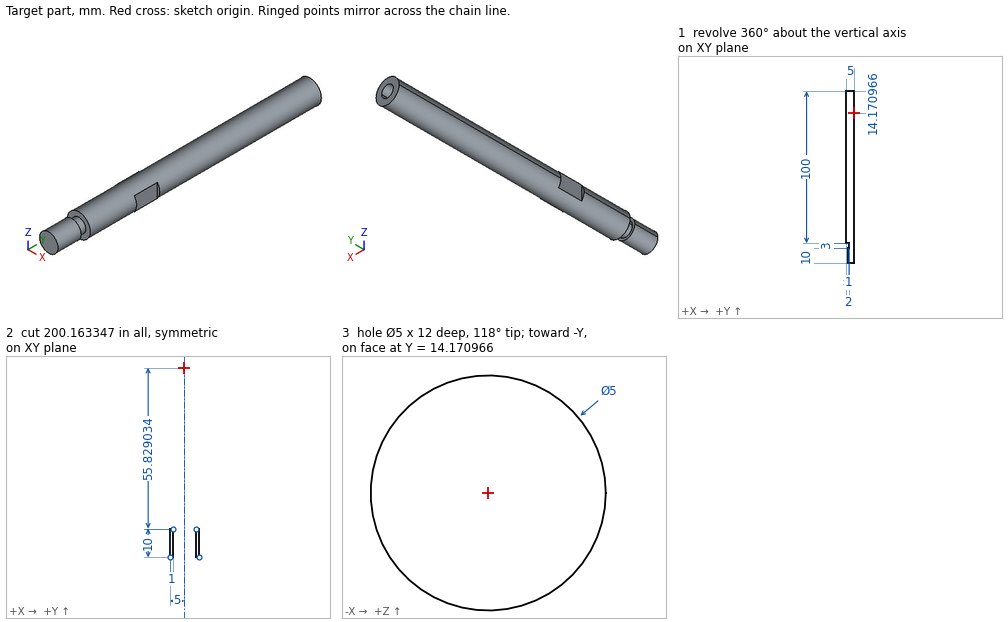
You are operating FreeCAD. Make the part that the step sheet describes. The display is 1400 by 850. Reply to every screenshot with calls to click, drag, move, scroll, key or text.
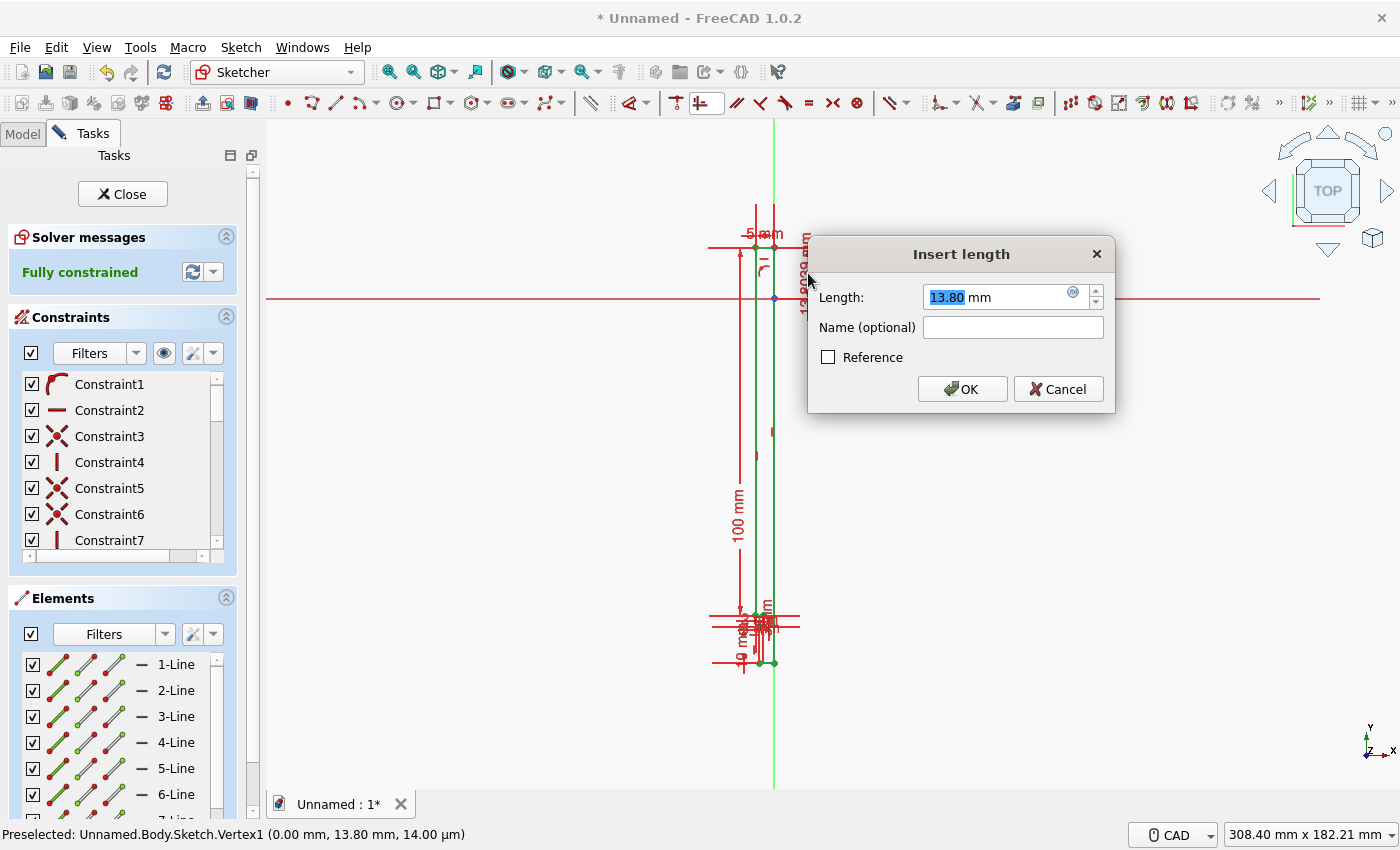
text(14.170966)
key(Return)
key(Escape)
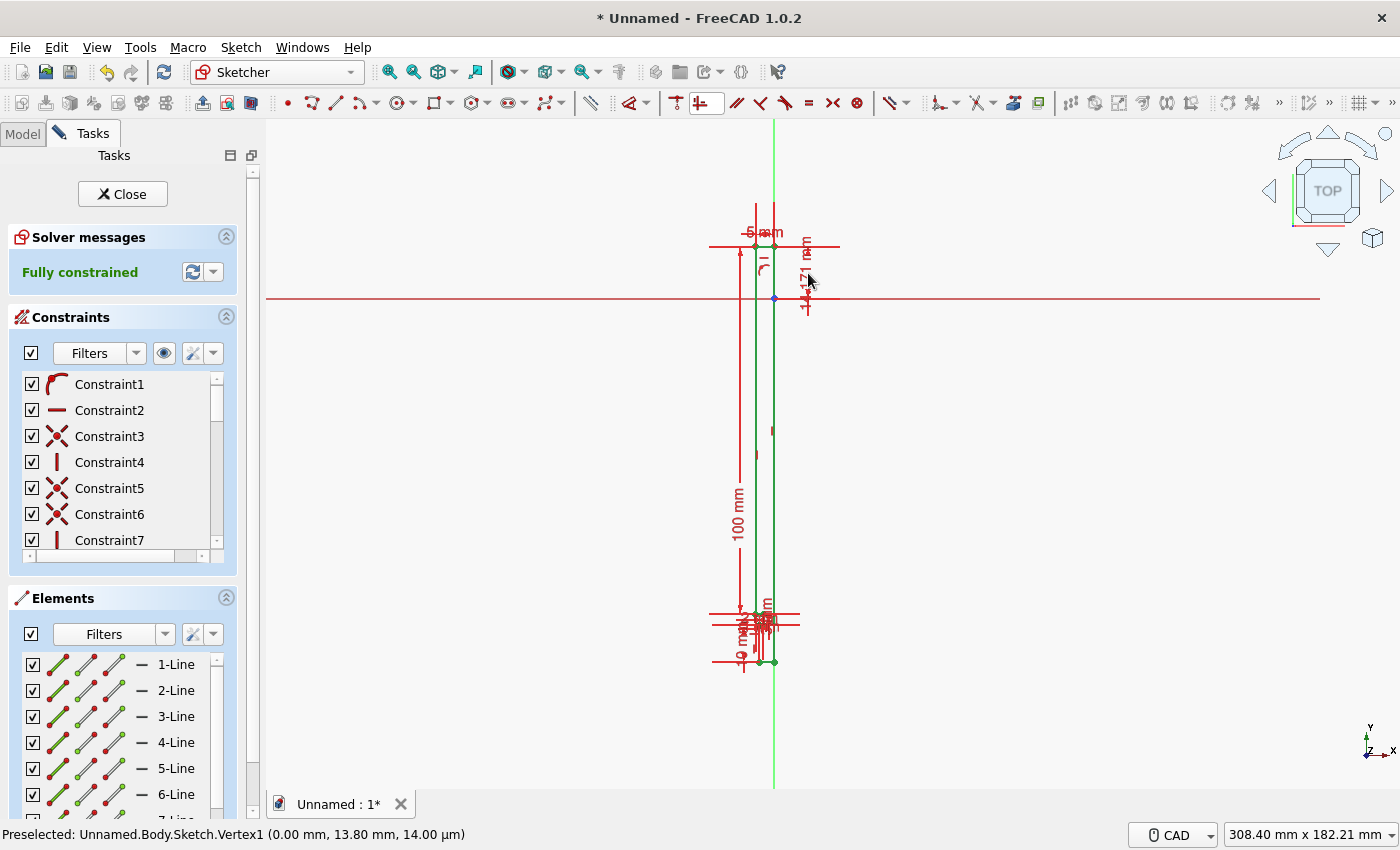
click(123, 194)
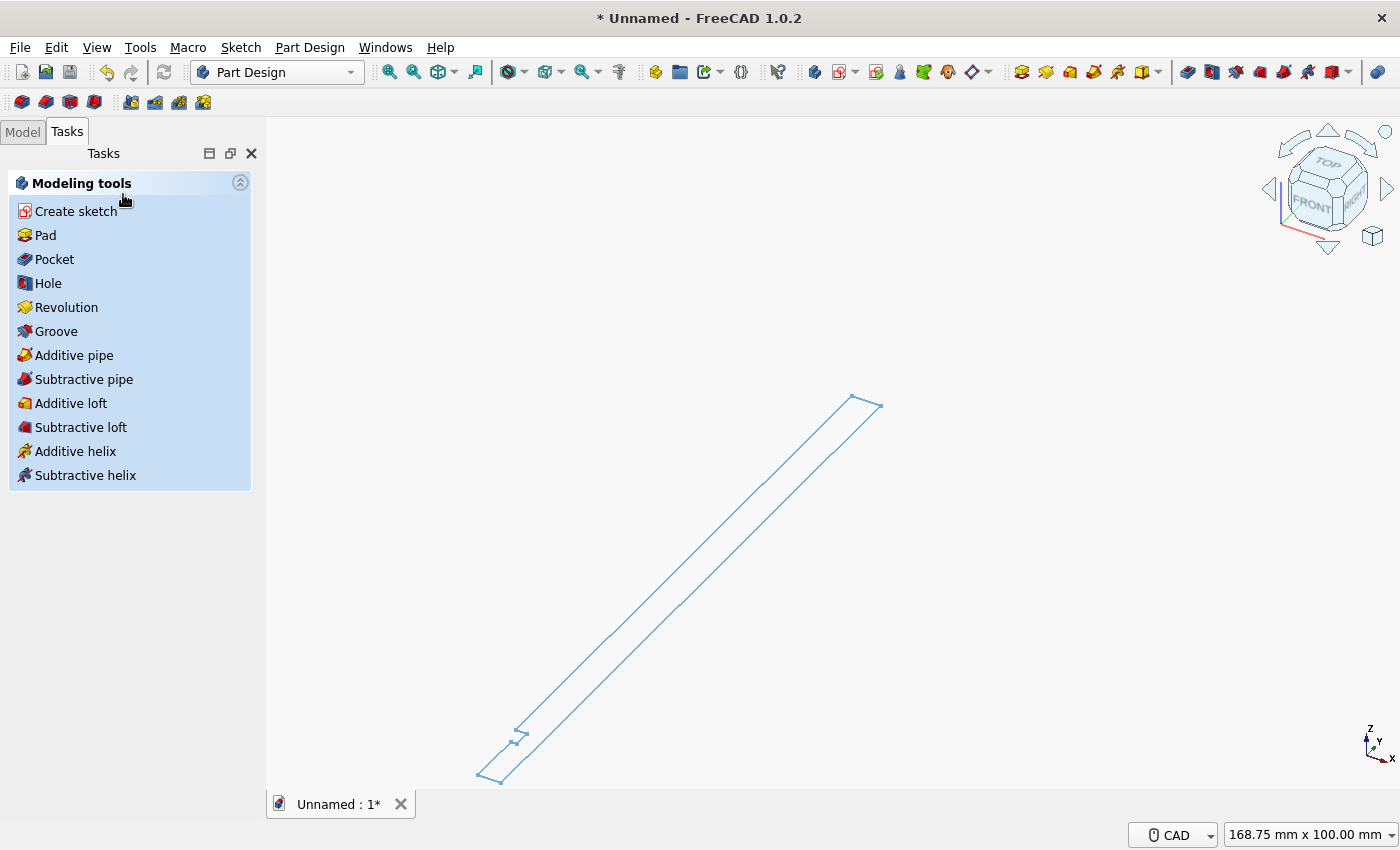
click(1046, 72)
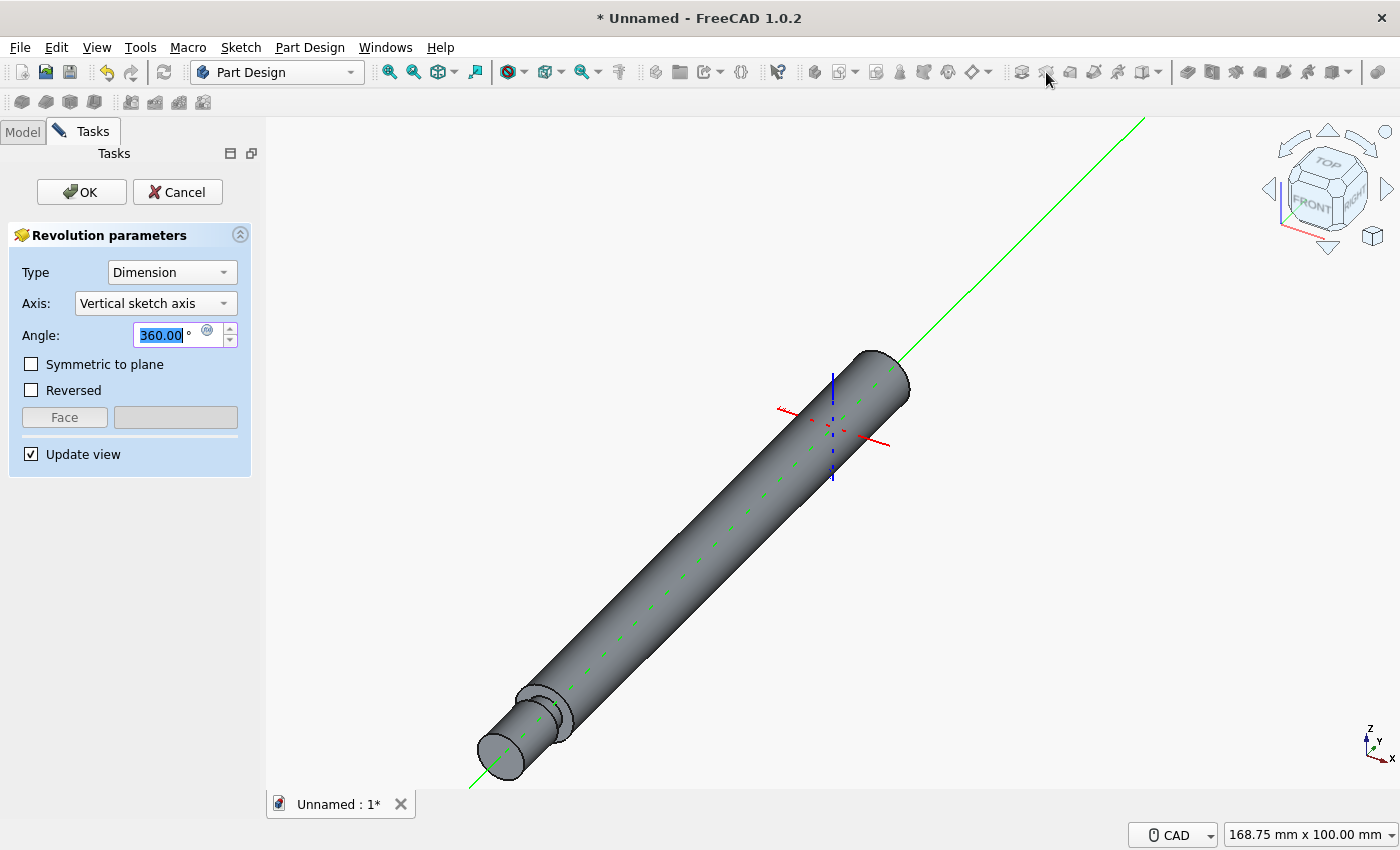
click(82, 192)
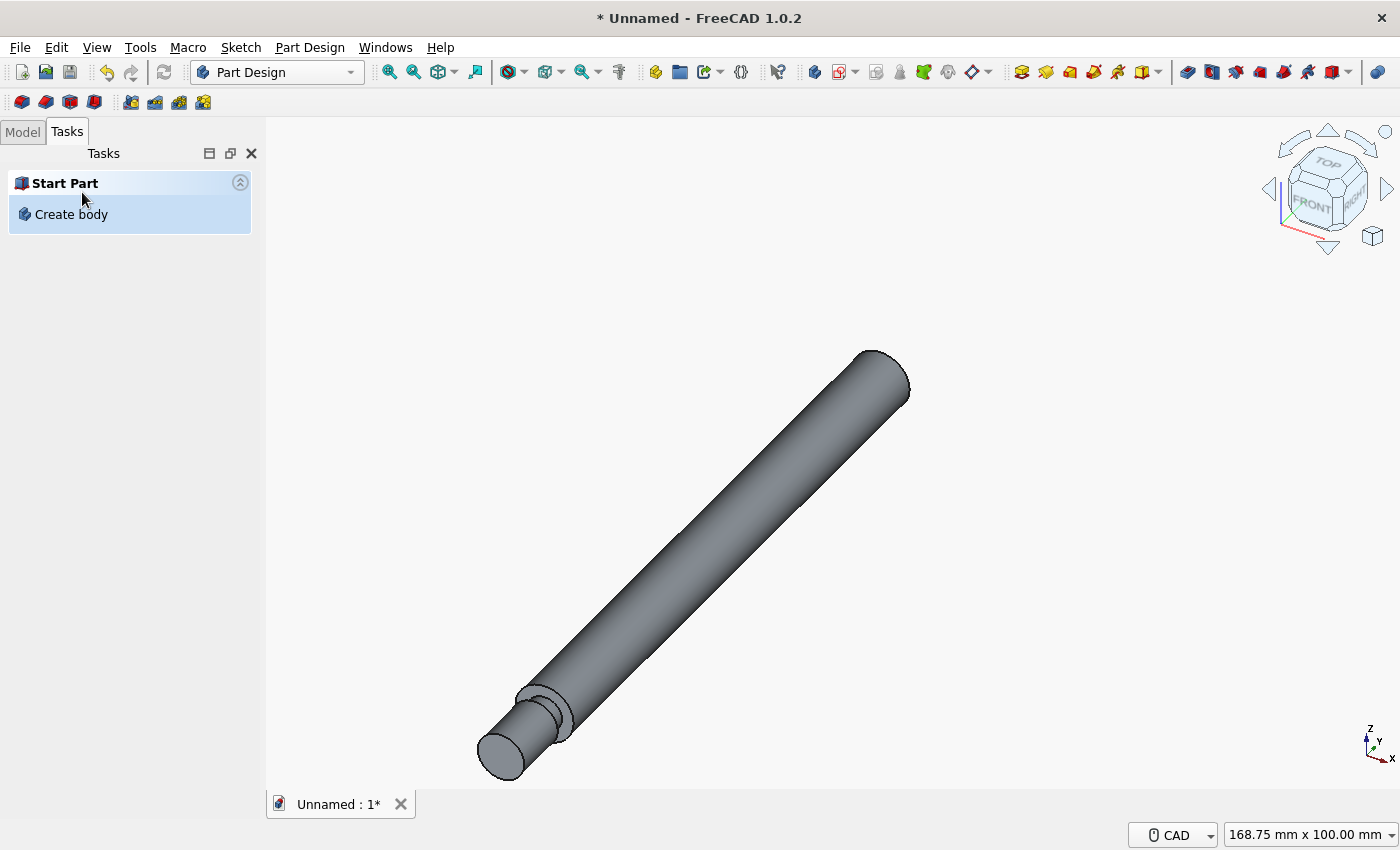
click(390, 72)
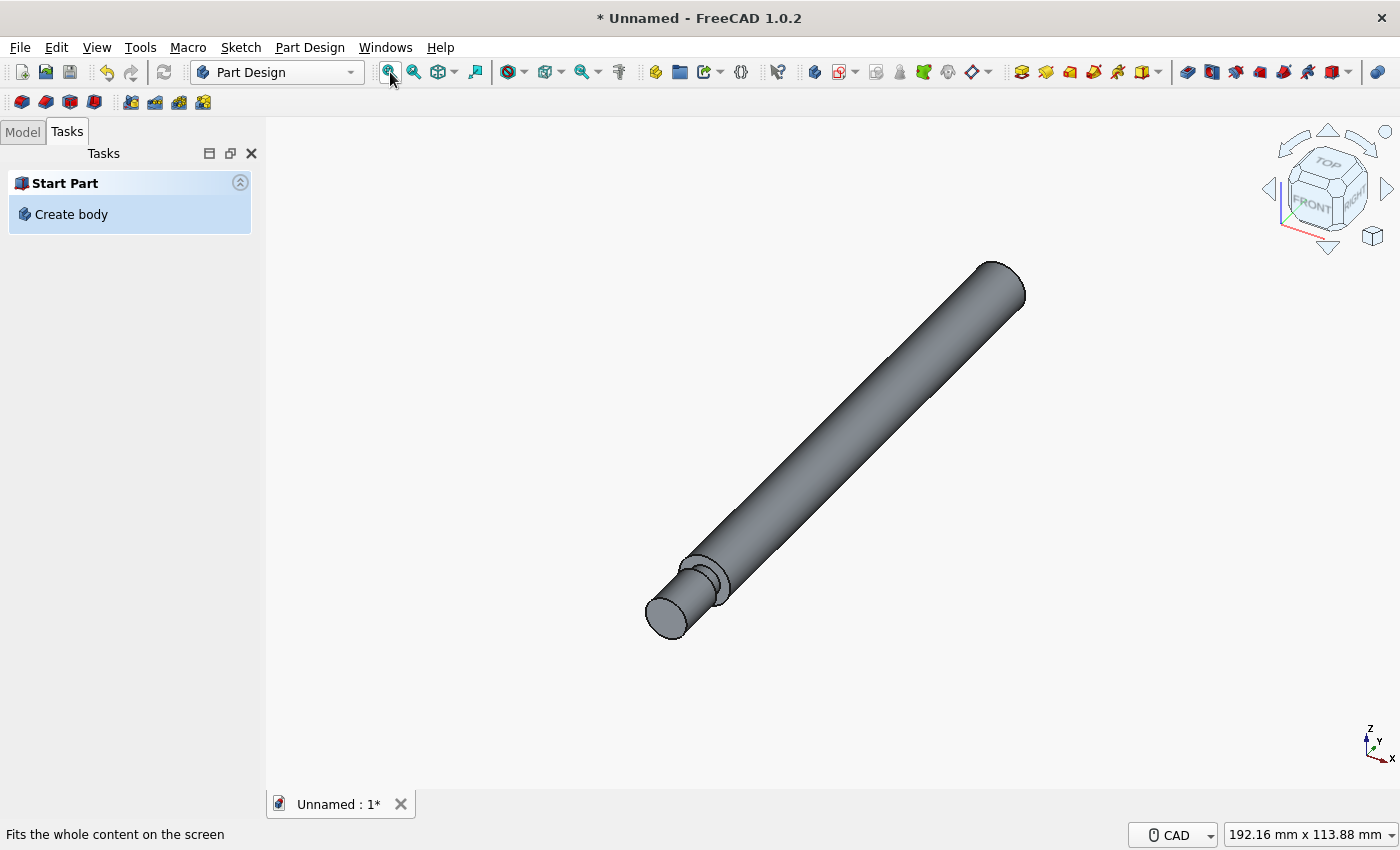
click(840, 72)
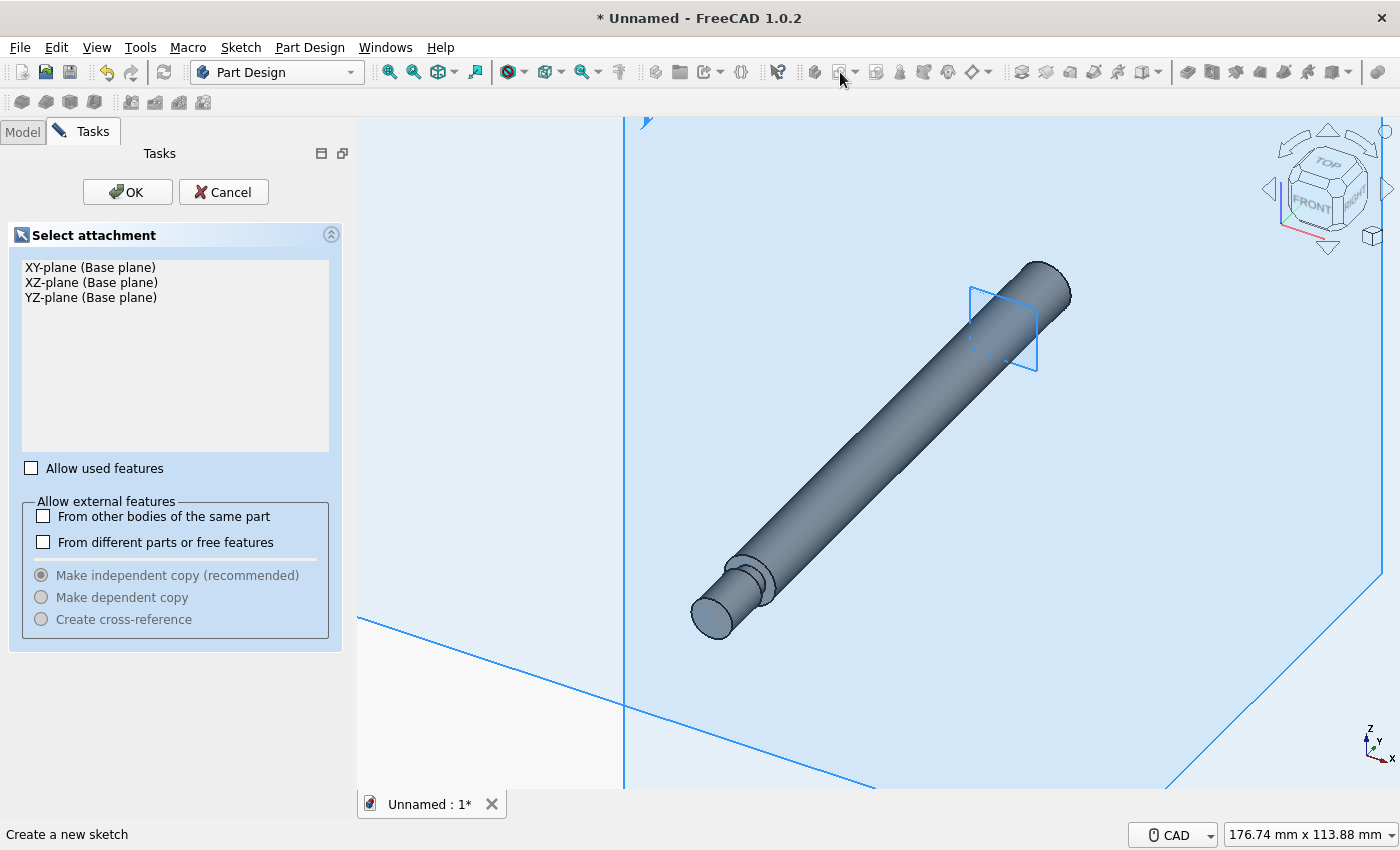
click(82, 268)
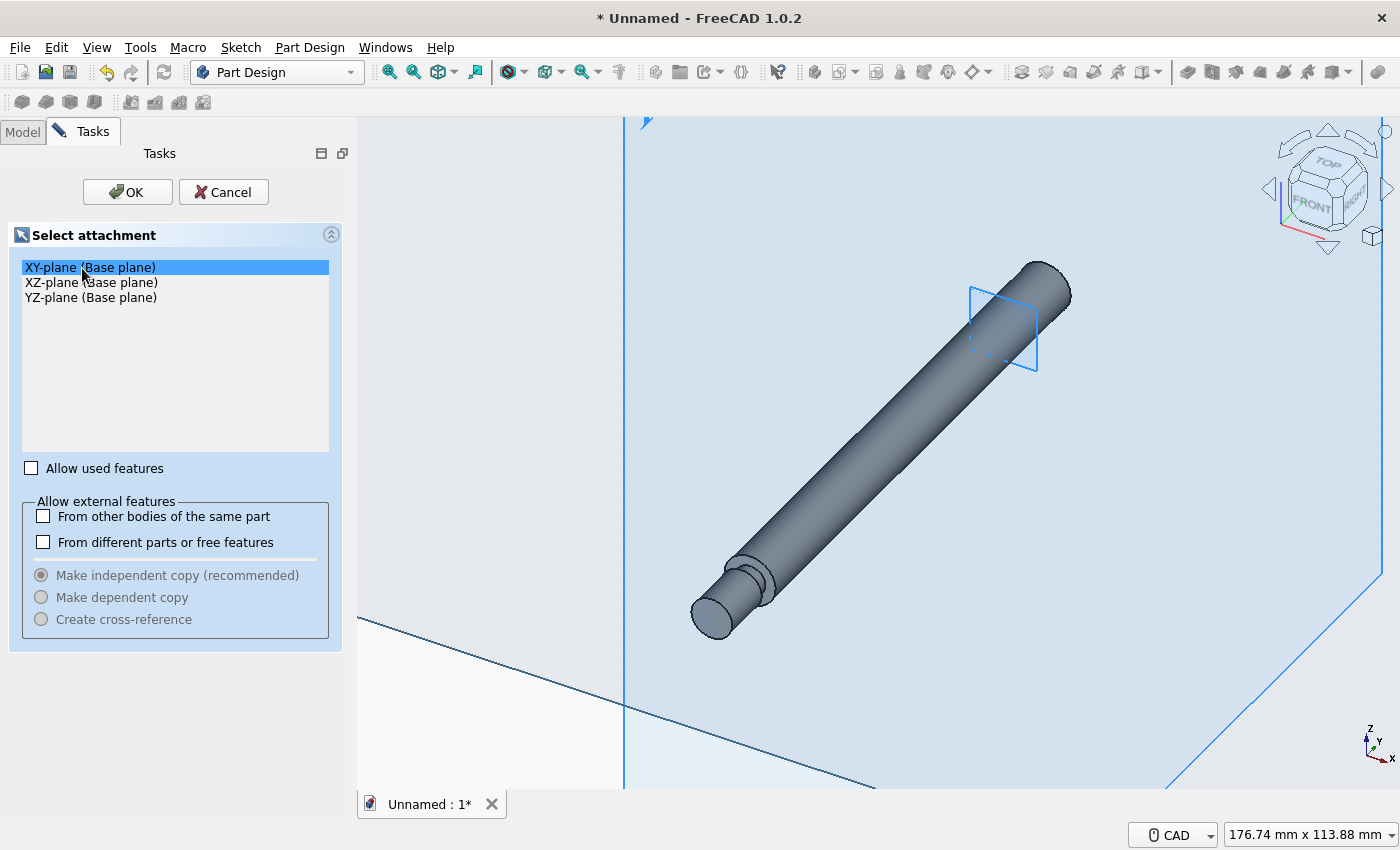
click(128, 192)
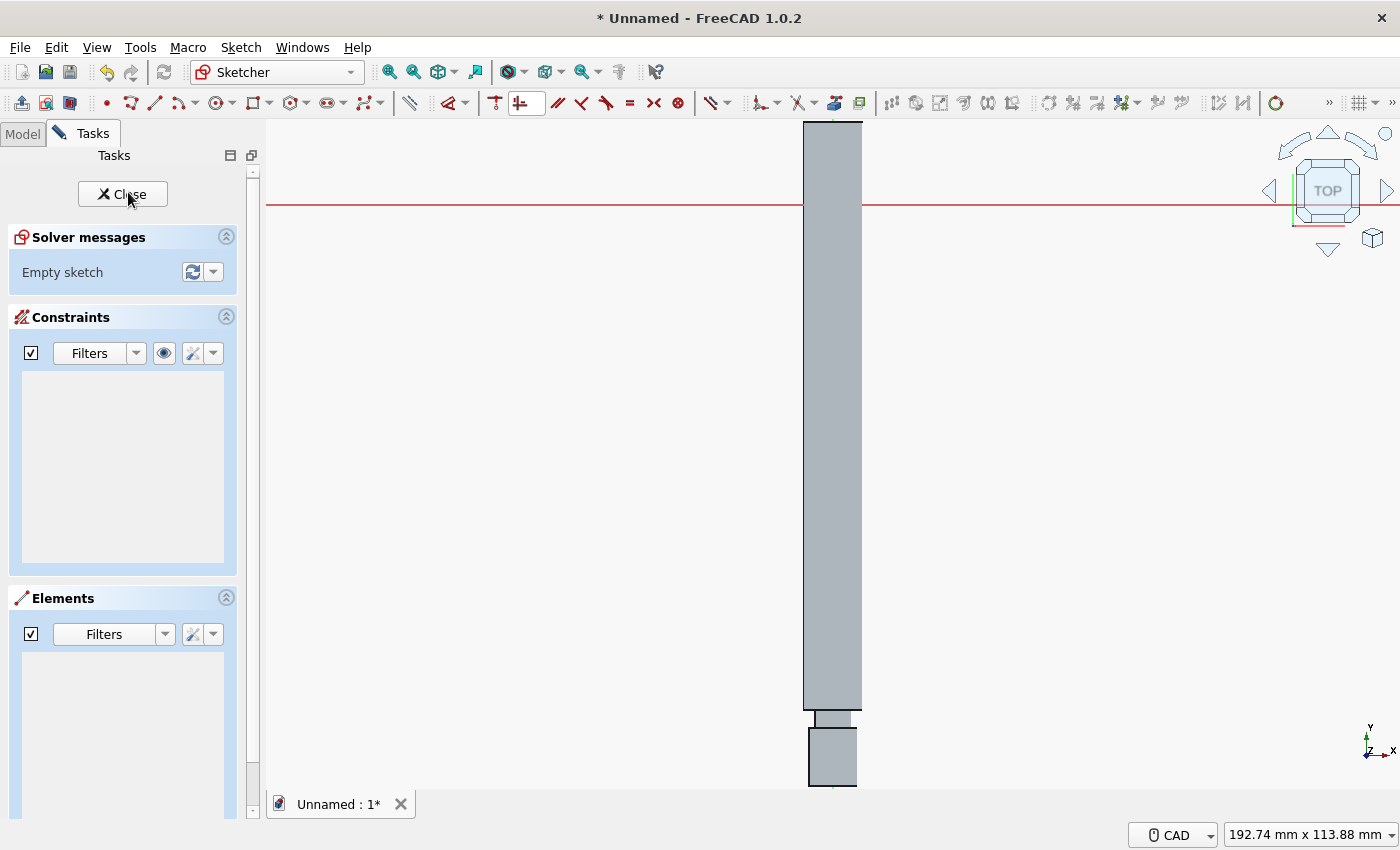
click(70, 104)